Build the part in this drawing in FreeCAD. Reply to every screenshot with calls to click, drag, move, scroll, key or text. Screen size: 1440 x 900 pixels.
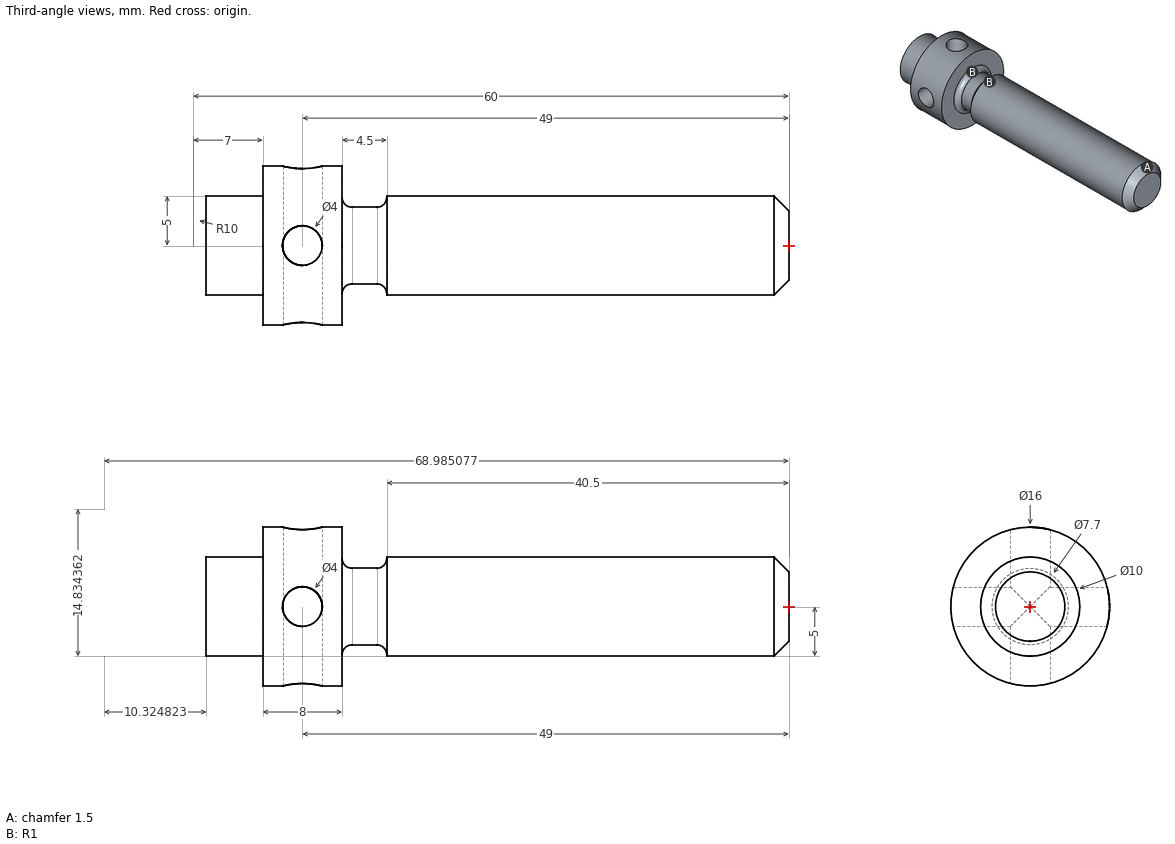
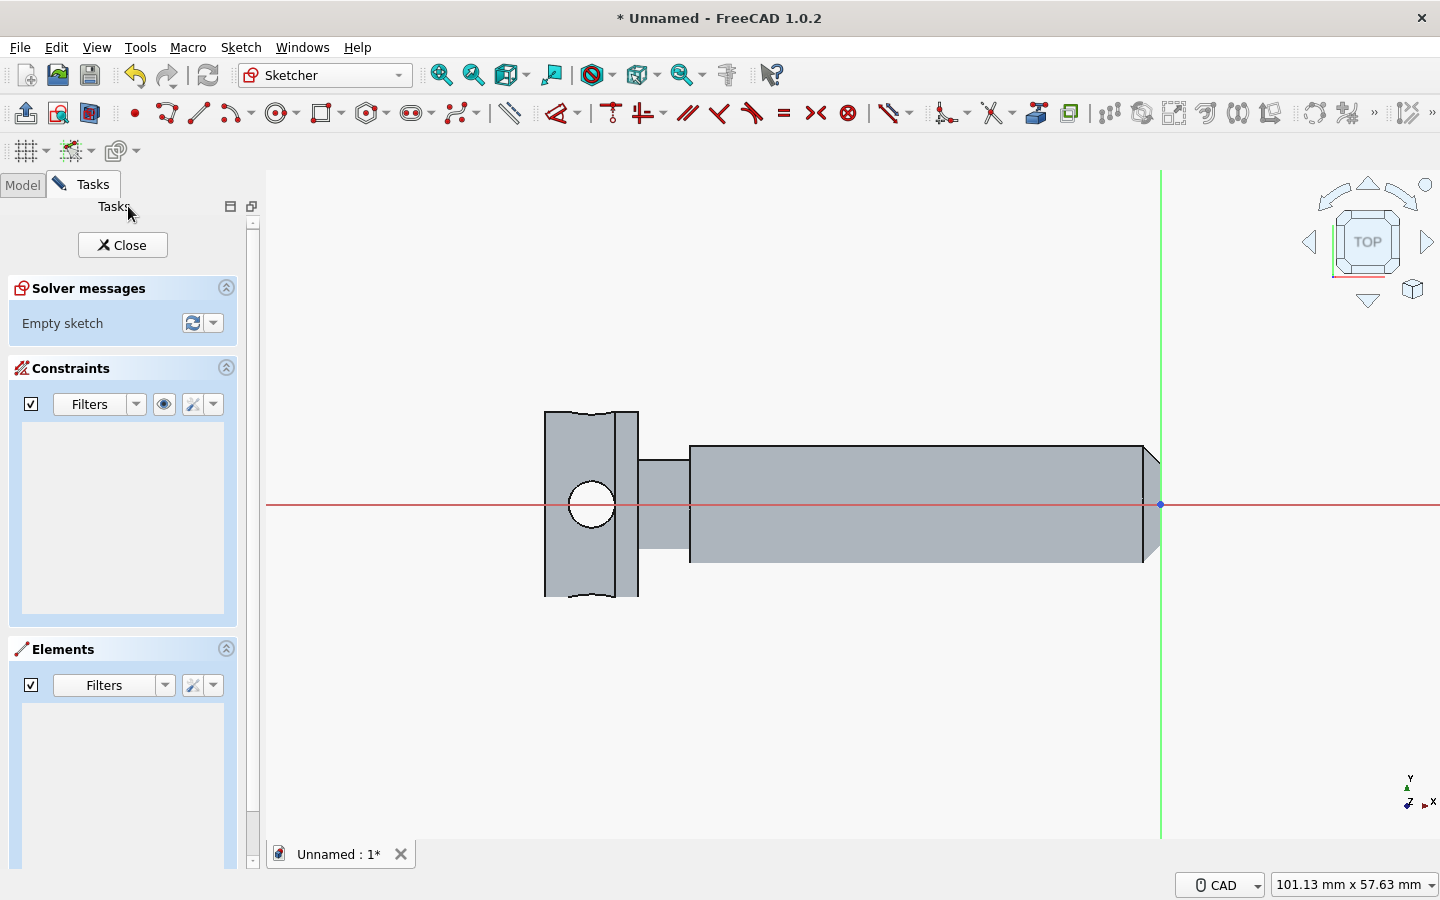
scroll(461, 471, up, 10)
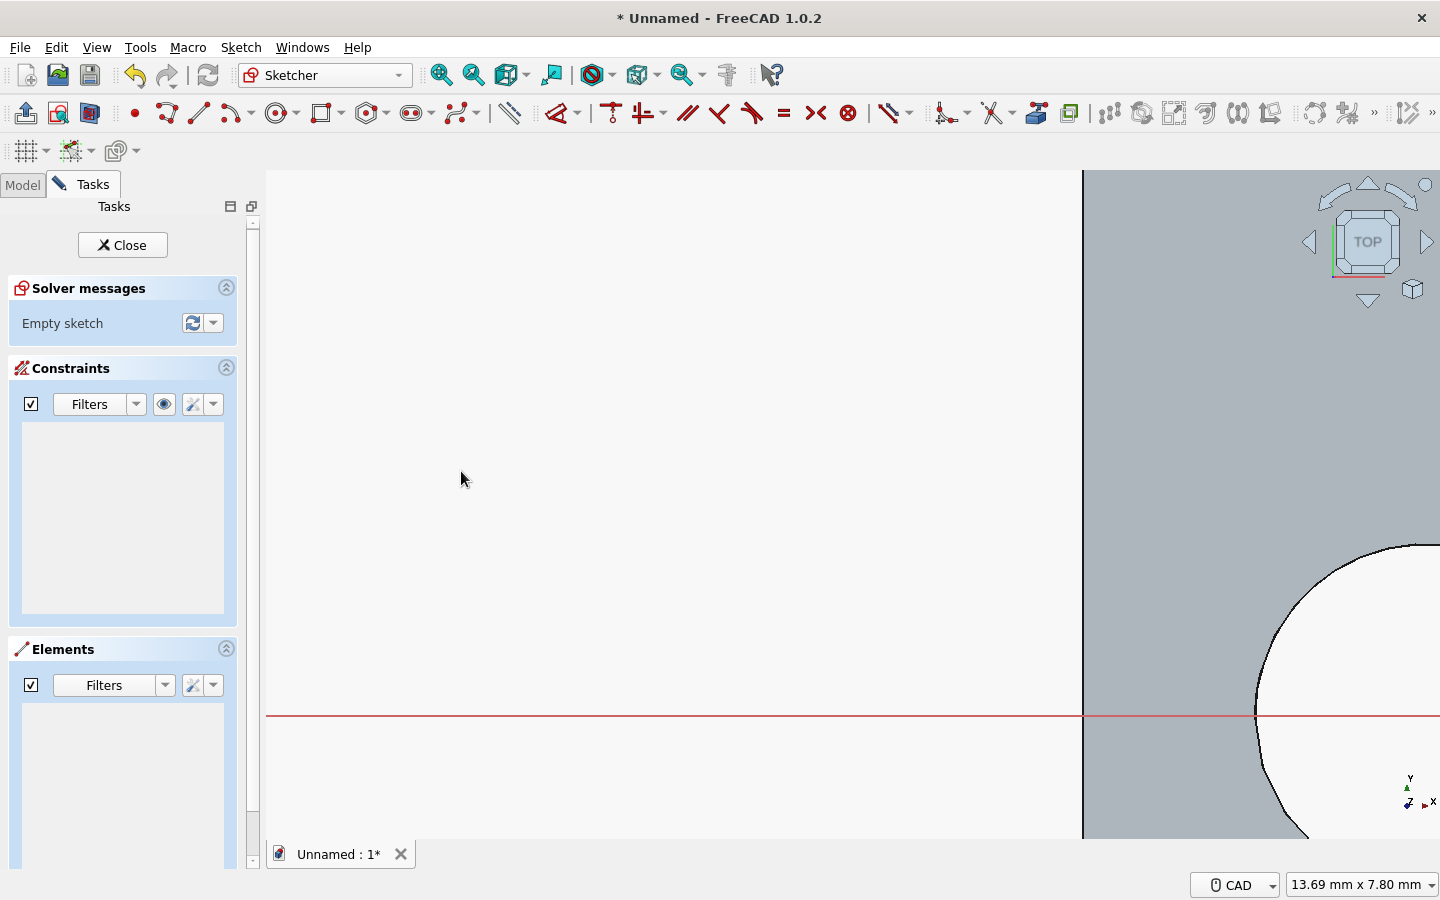
key(g)
key(m)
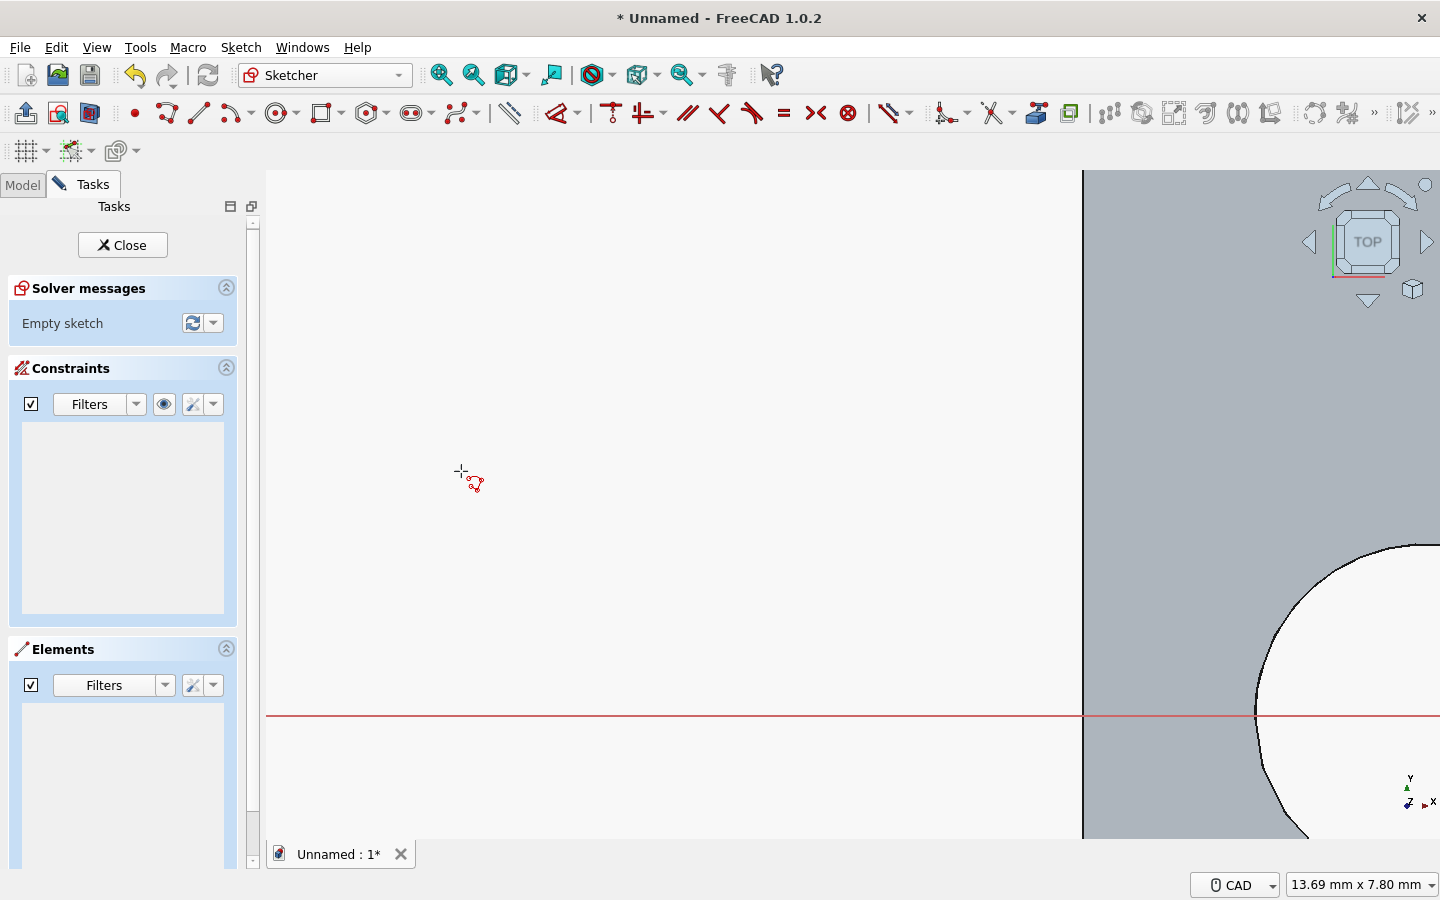
click(483, 716)
click(1083, 707)
click(1083, 287)
click(598, 287)
right_click(598, 287)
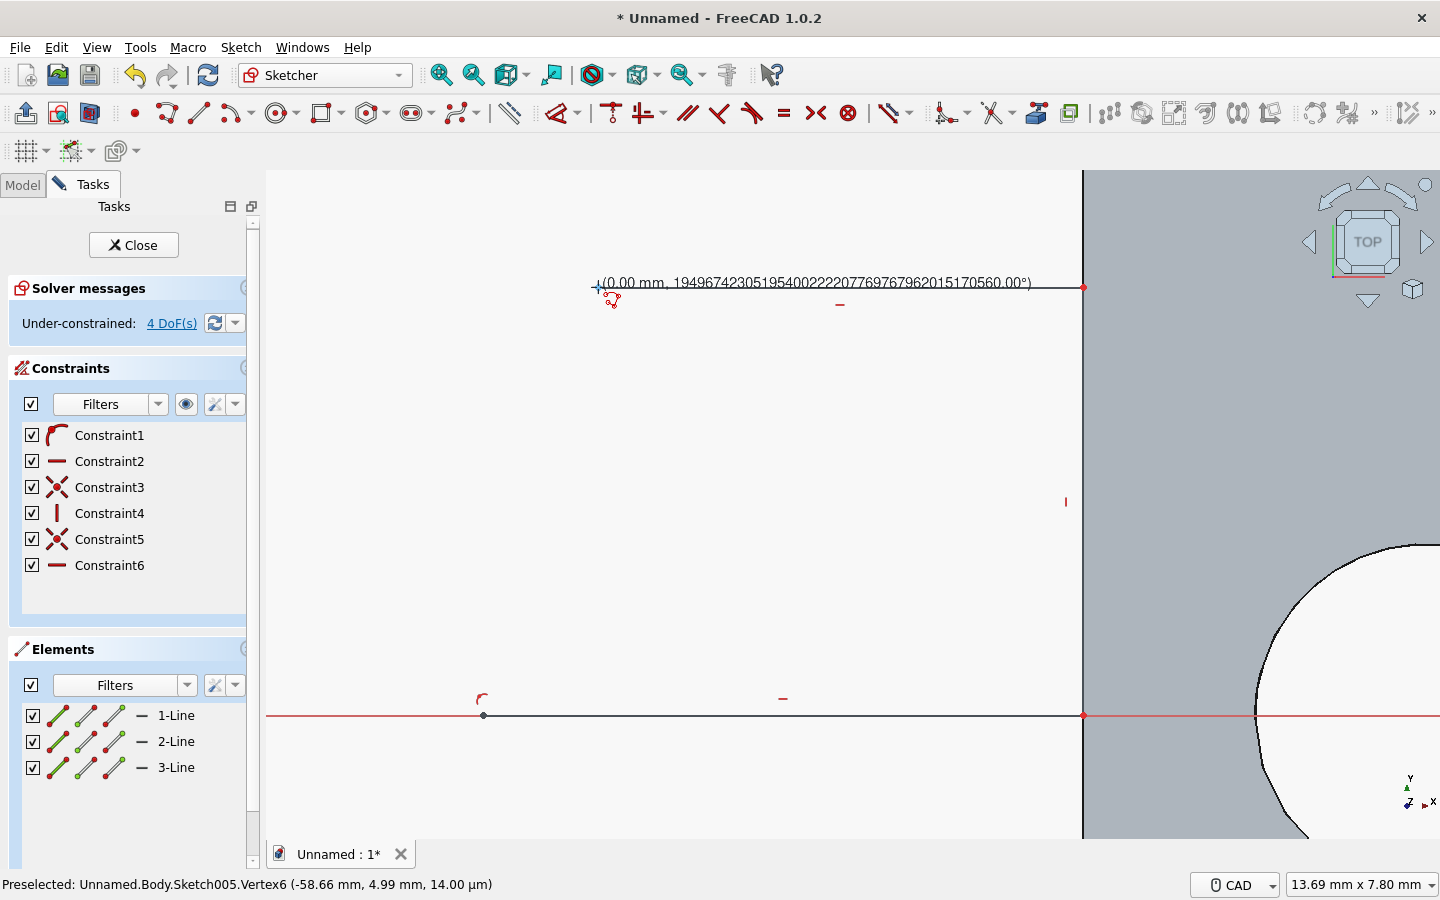
click(254, 114)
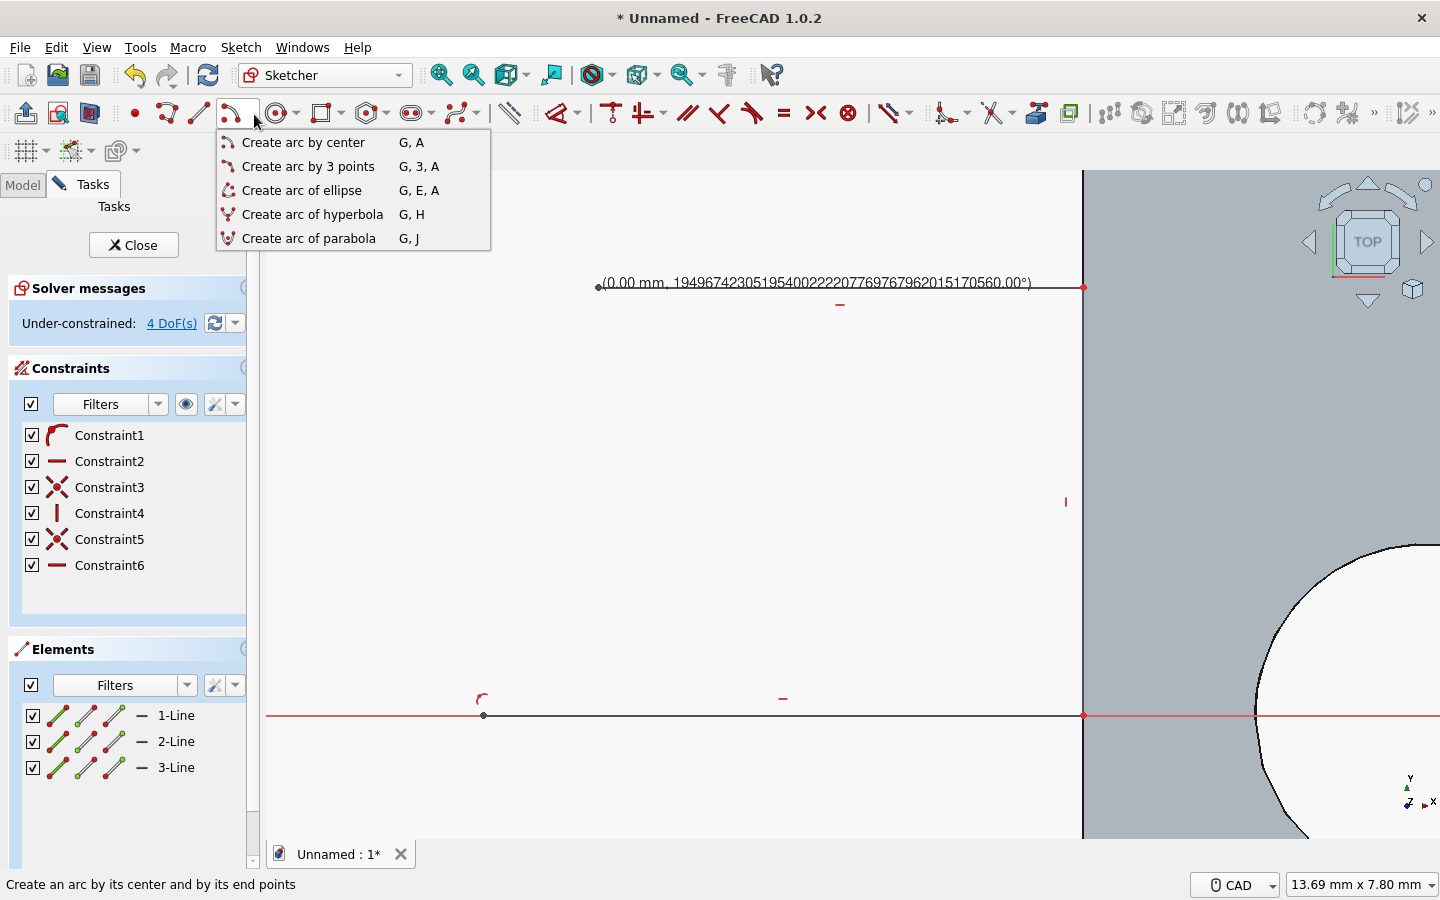
click(354, 166)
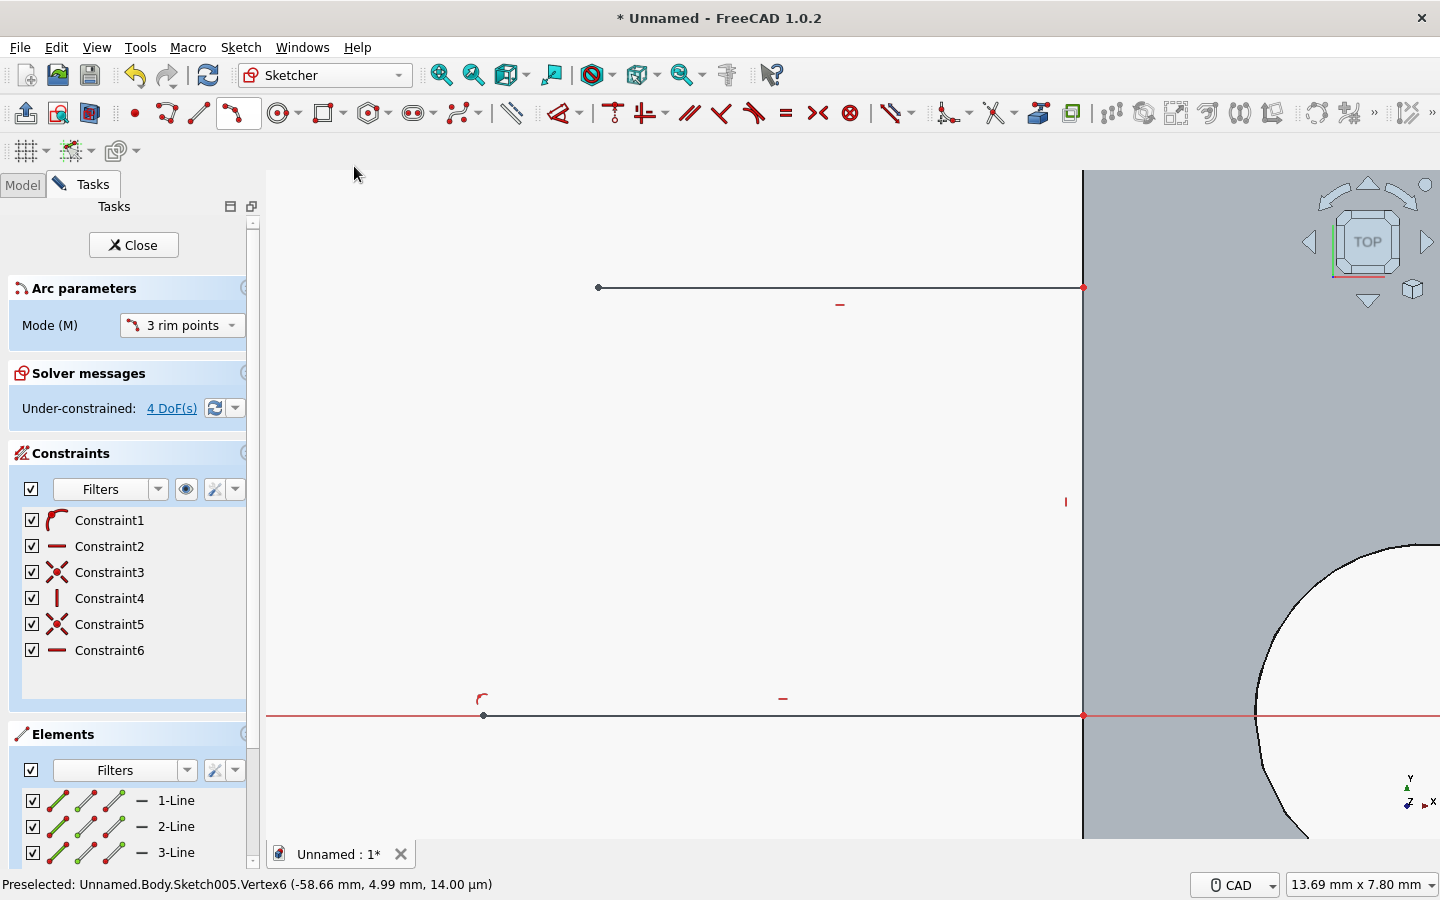
click(598, 288)
click(483, 716)
click(512, 494)
key(Escape)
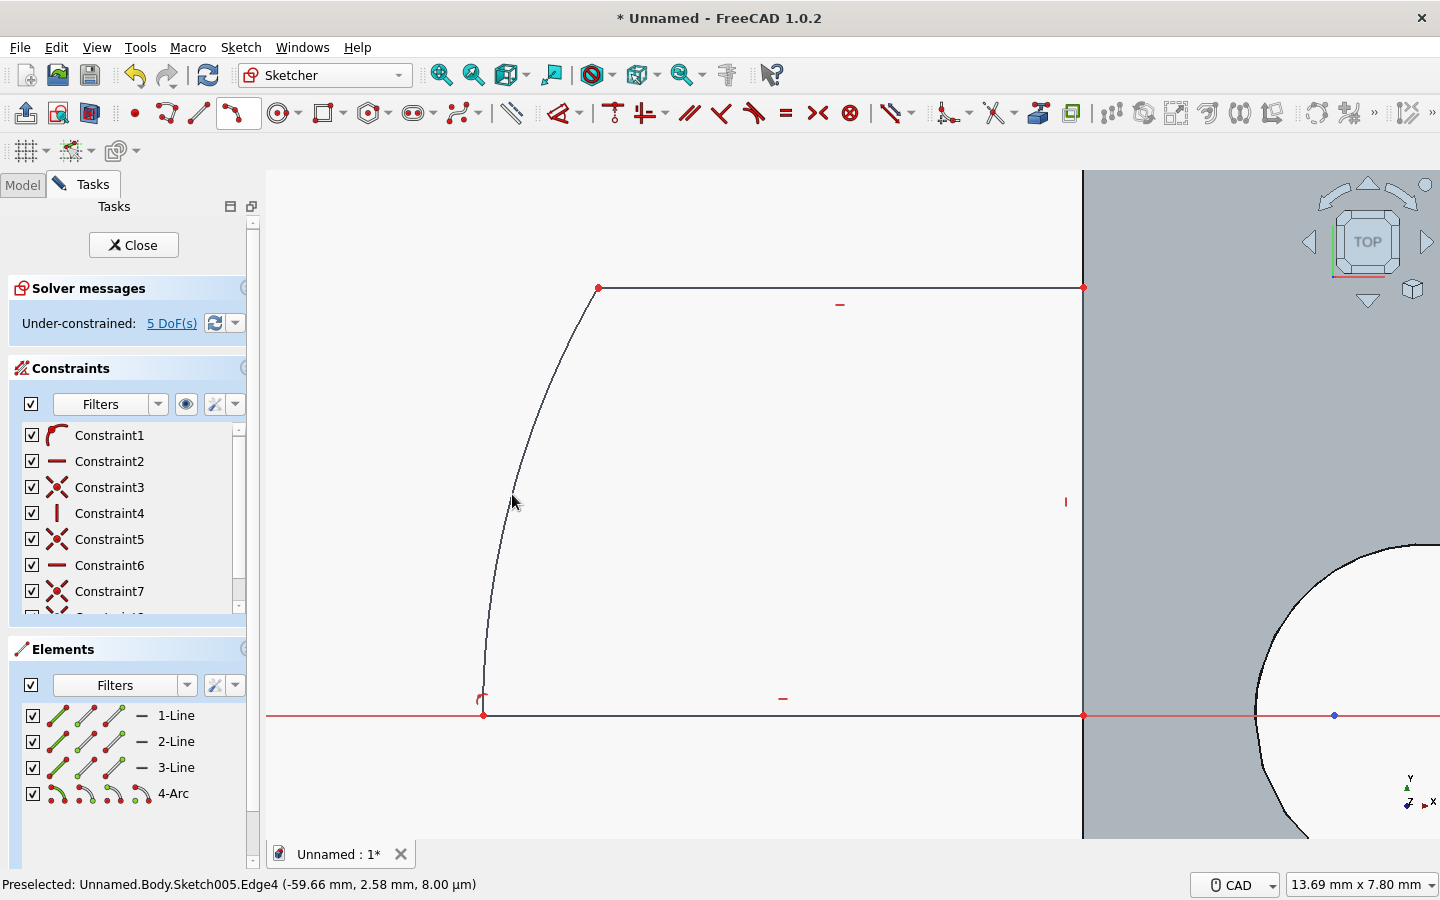
scroll(294, 519, down, 1)